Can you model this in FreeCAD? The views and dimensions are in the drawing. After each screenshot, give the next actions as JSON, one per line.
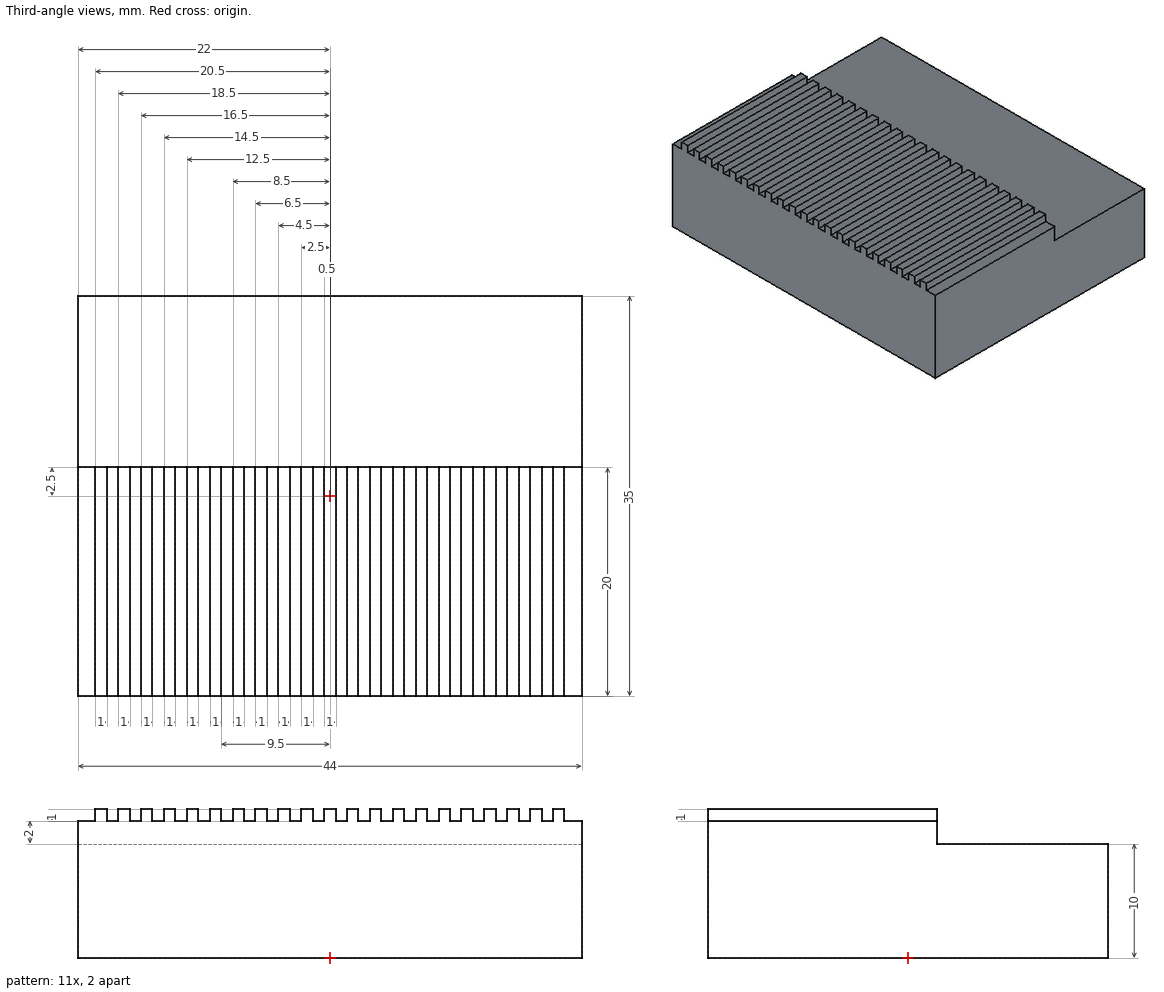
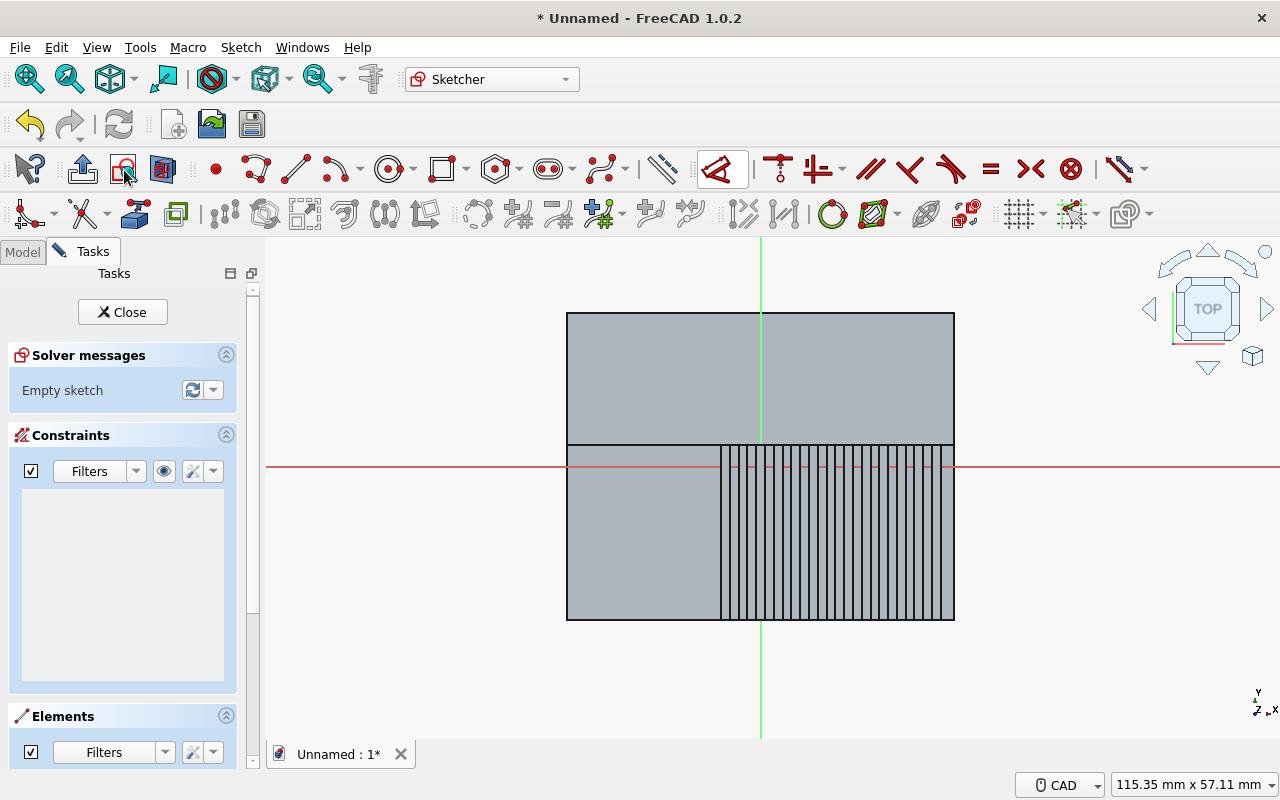
{"action": "left_click", "coordinate": [164, 170]}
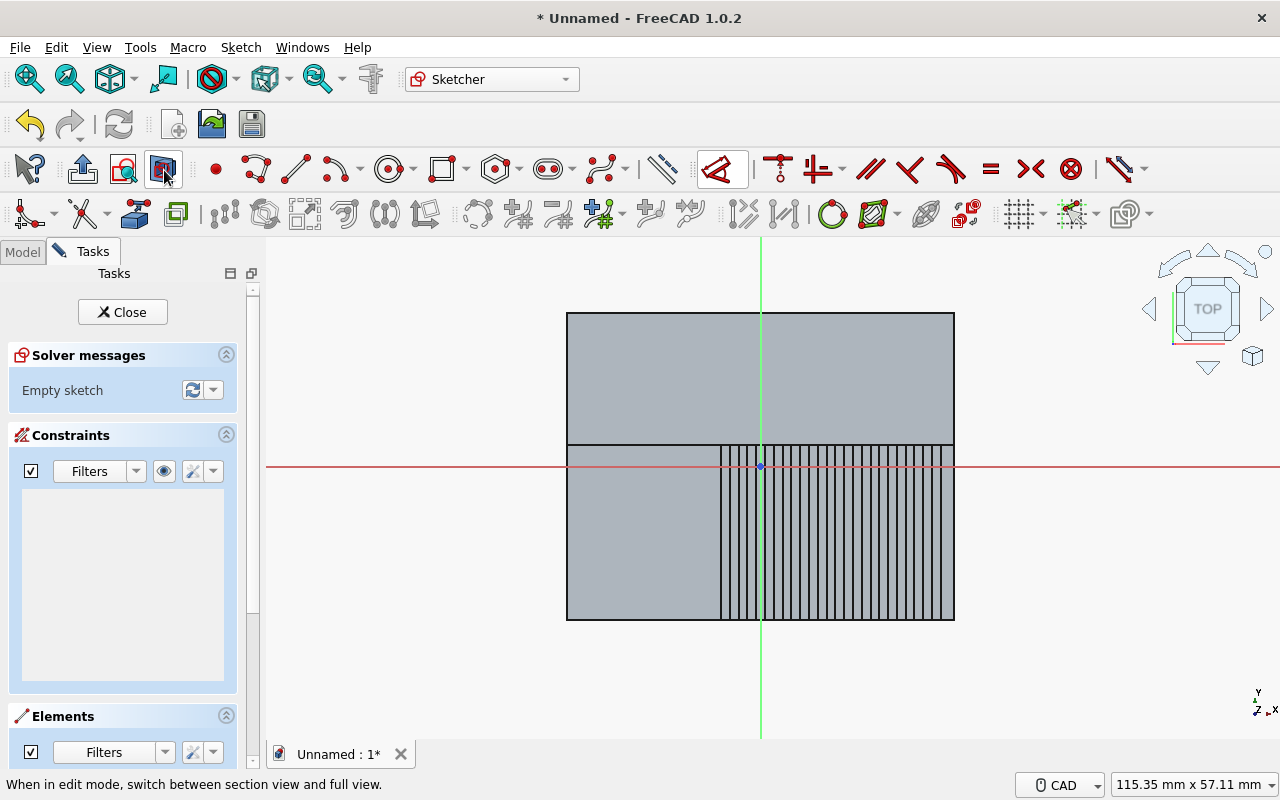
{"action": "scroll", "coordinate": [766, 587], "scroll_direction": "up", "scroll_amount": 3}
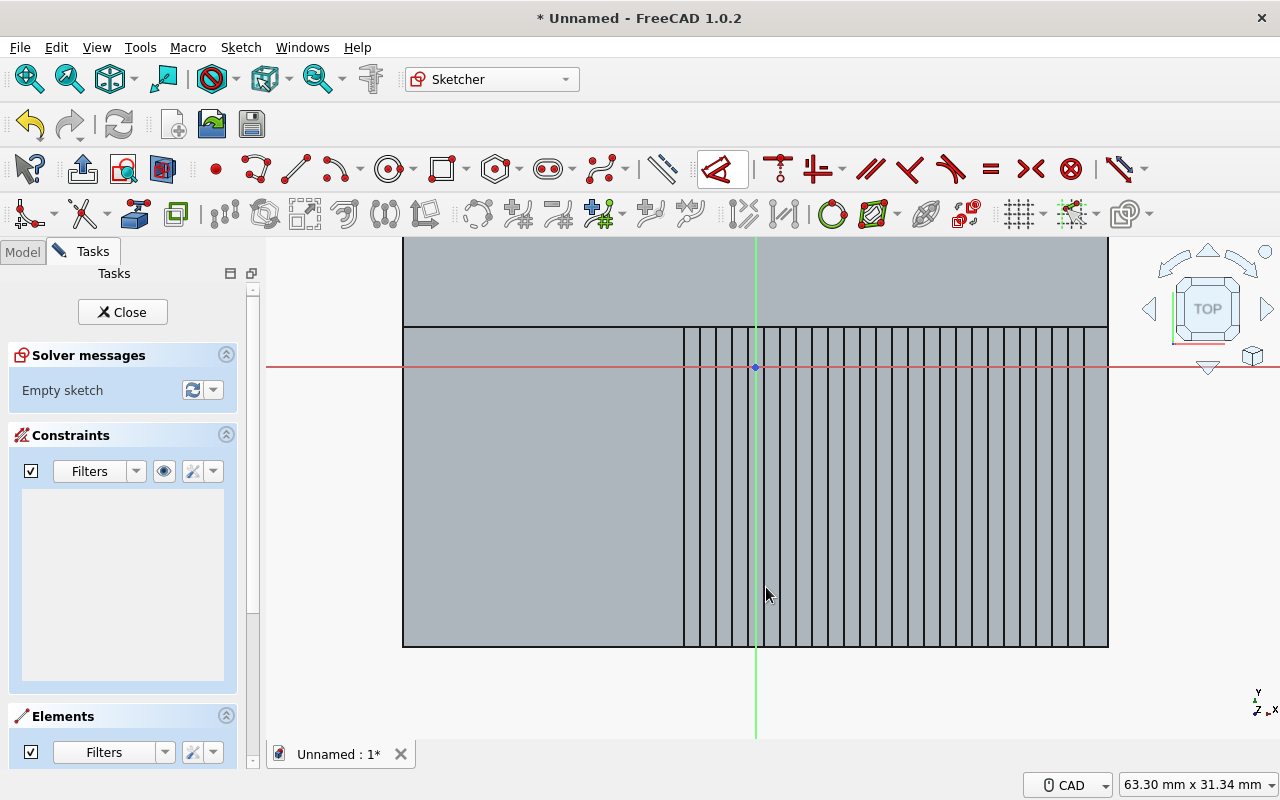
{"action": "left_click", "coordinate": [442, 170]}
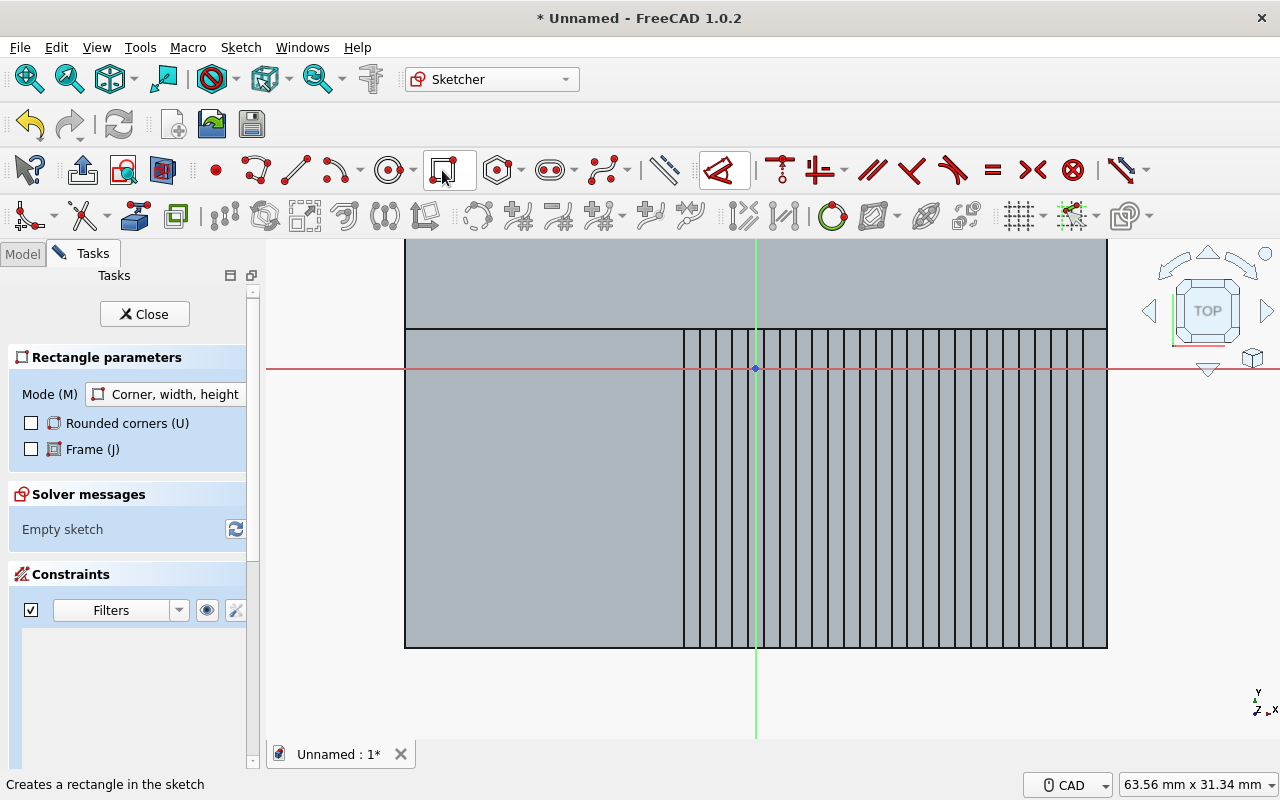
{"action": "left_click", "coordinate": [652, 329]}
{"action": "mouse_move", "coordinate": [668, 648]}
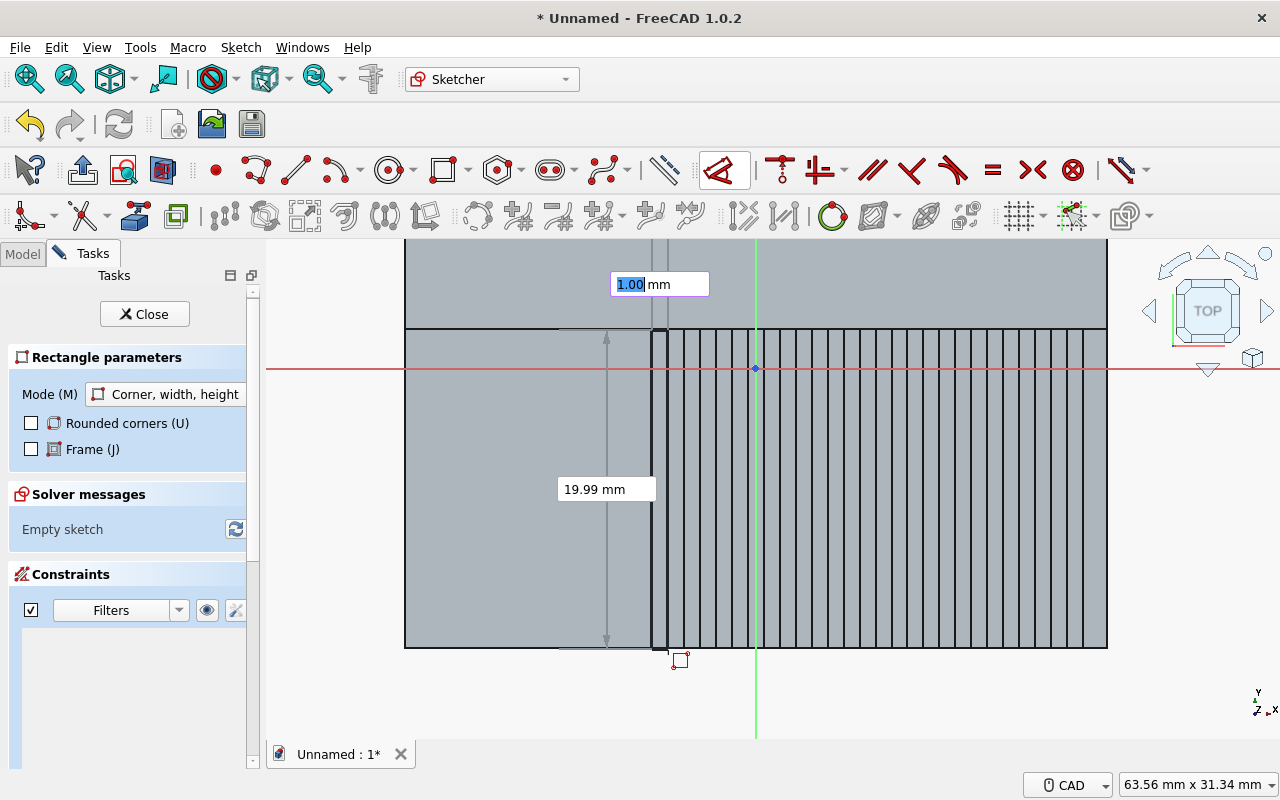
{"action": "type", "text": "1"}
{"action": "key", "text": "Tab"}
{"action": "type", "text": "20"}
{"action": "key", "text": "Return"}
{"action": "key", "text": "Escape"}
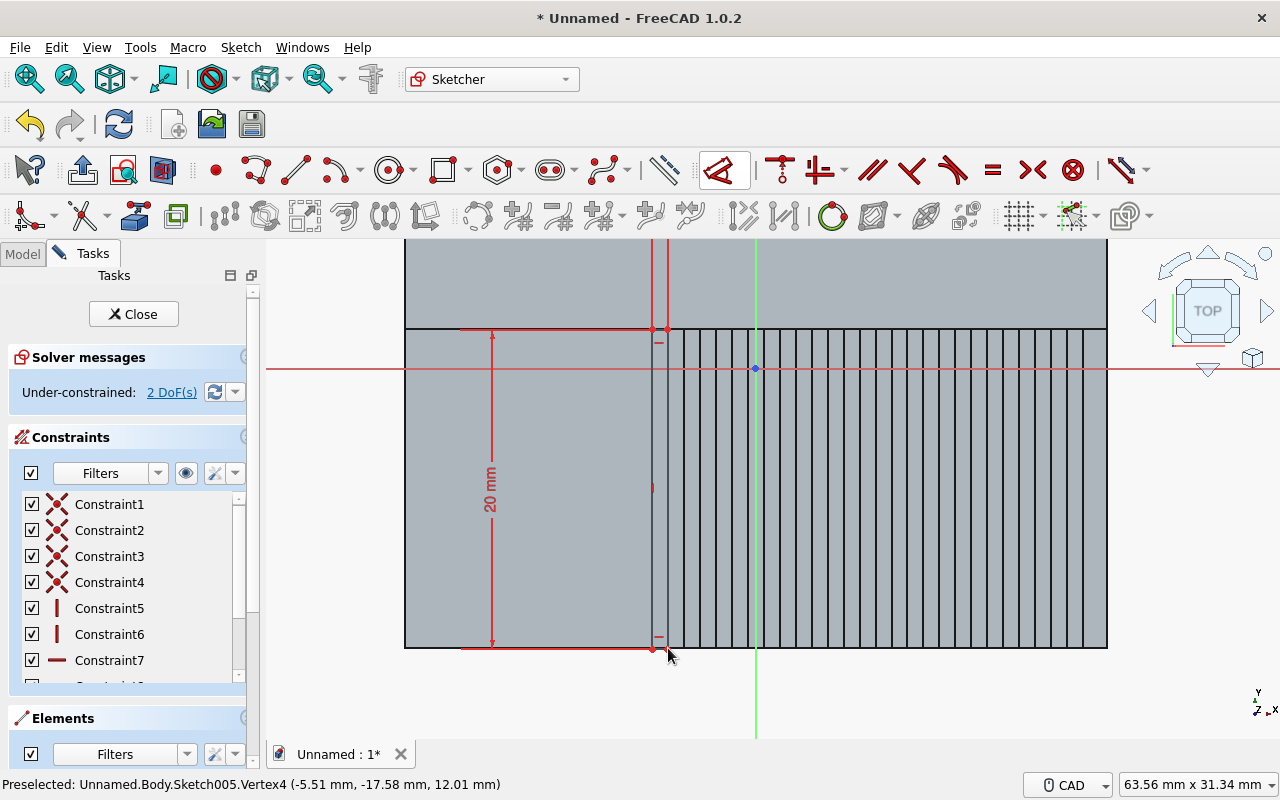
{"action": "left_click", "coordinate": [652, 330]}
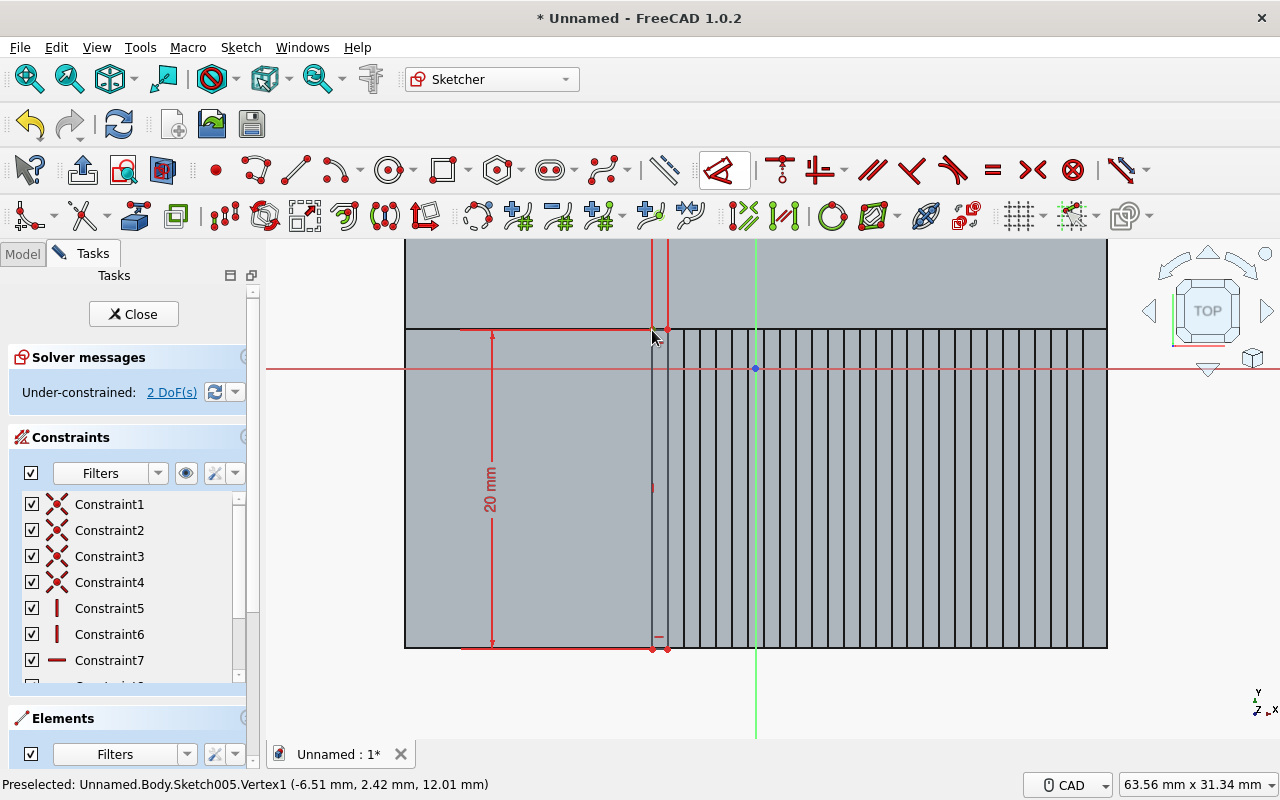
{"action": "key", "text": "l"}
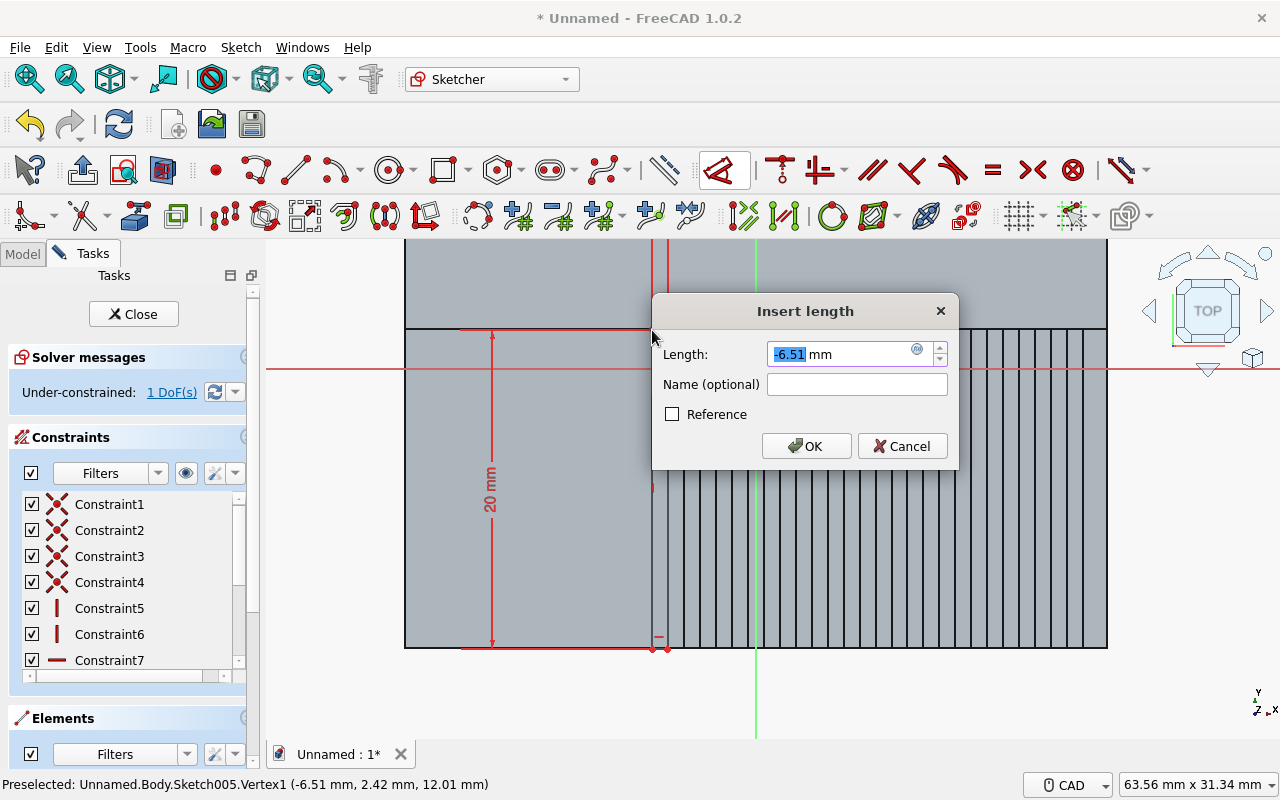
{"action": "type", "text": "-6.5"}
{"action": "key", "text": "Return"}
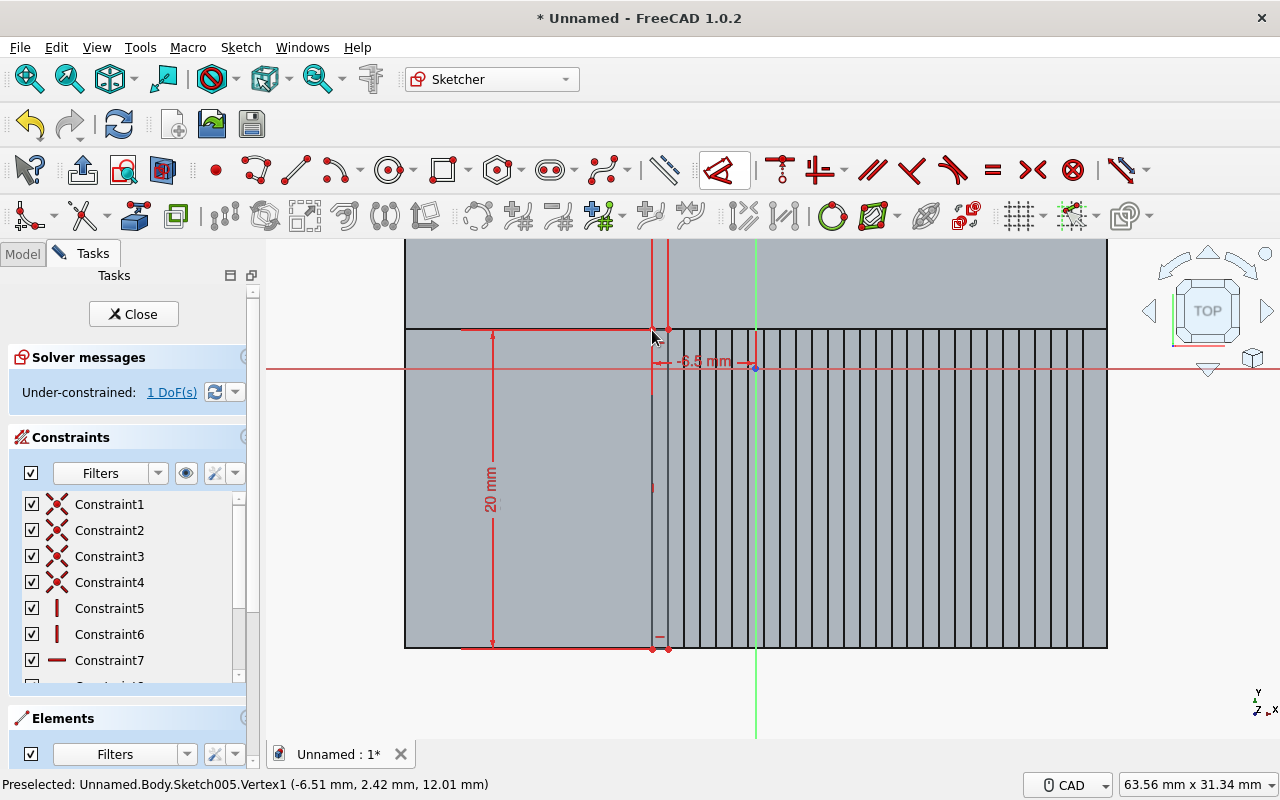
{"action": "left_click", "coordinate": [652, 330]}